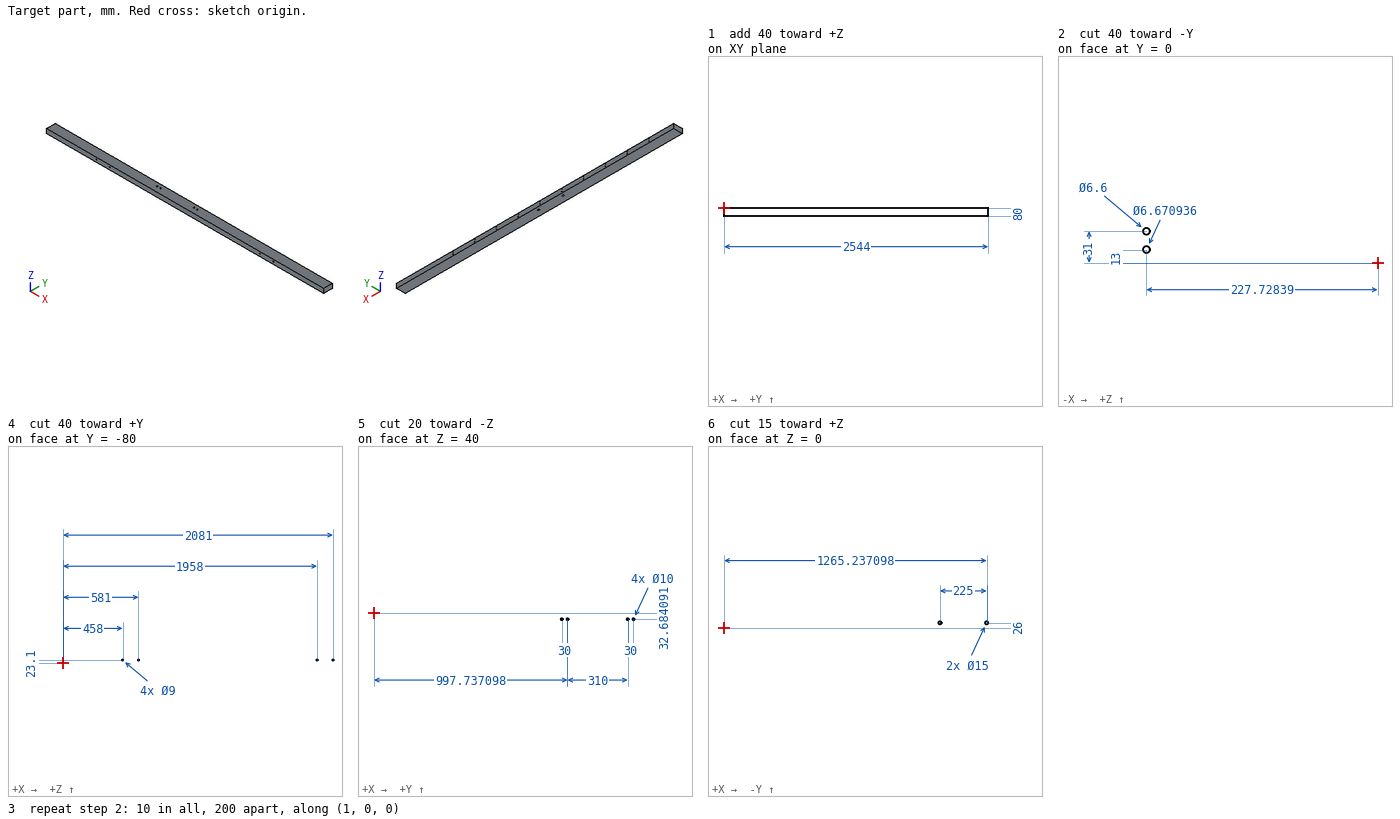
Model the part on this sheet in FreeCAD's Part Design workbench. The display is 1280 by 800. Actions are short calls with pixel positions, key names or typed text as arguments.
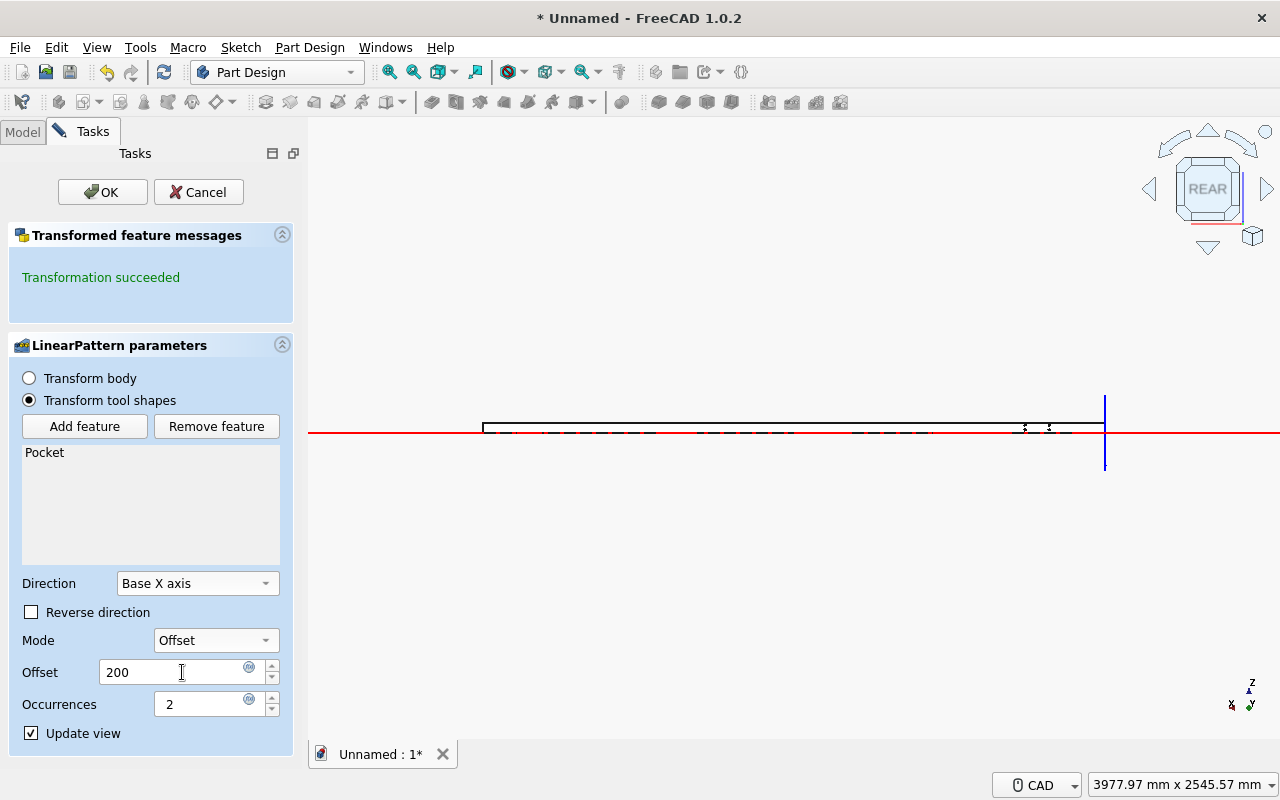
triple_click(209, 704)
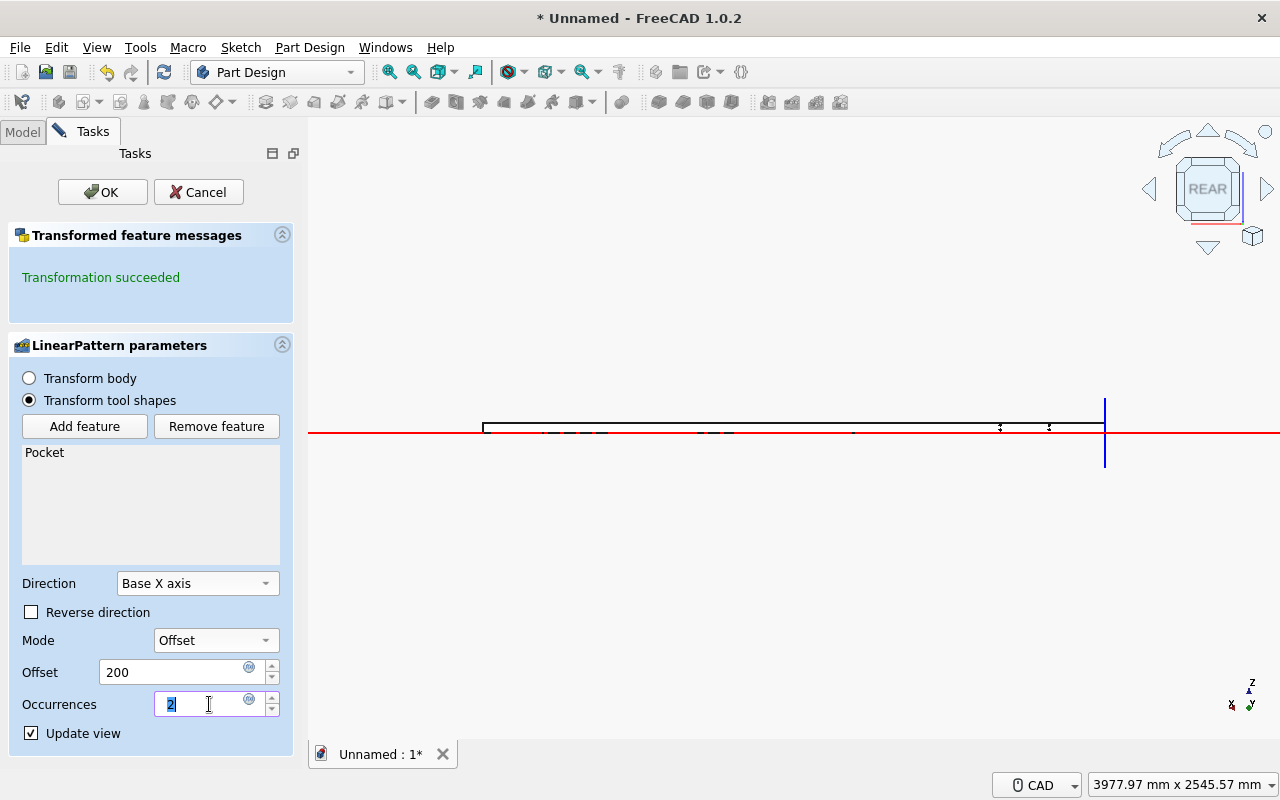
text(10)
key(Tab)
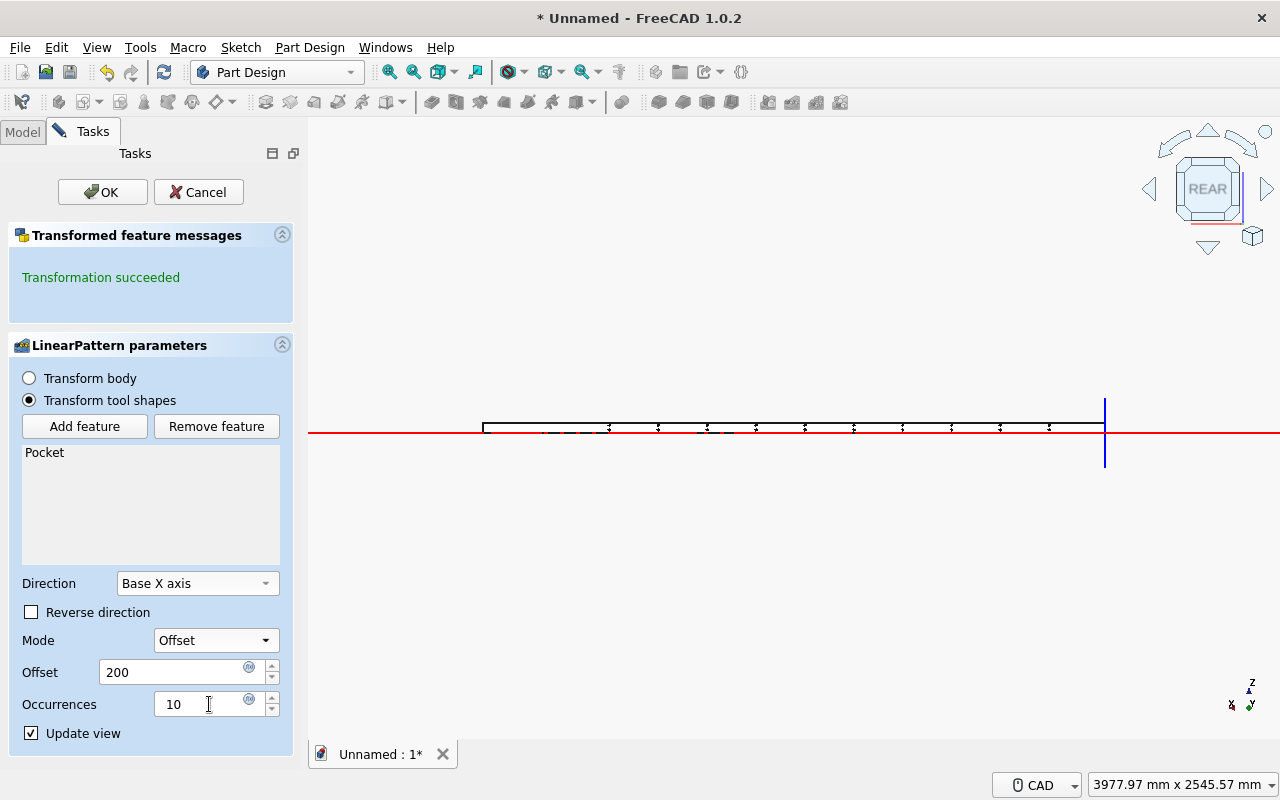
click(103, 192)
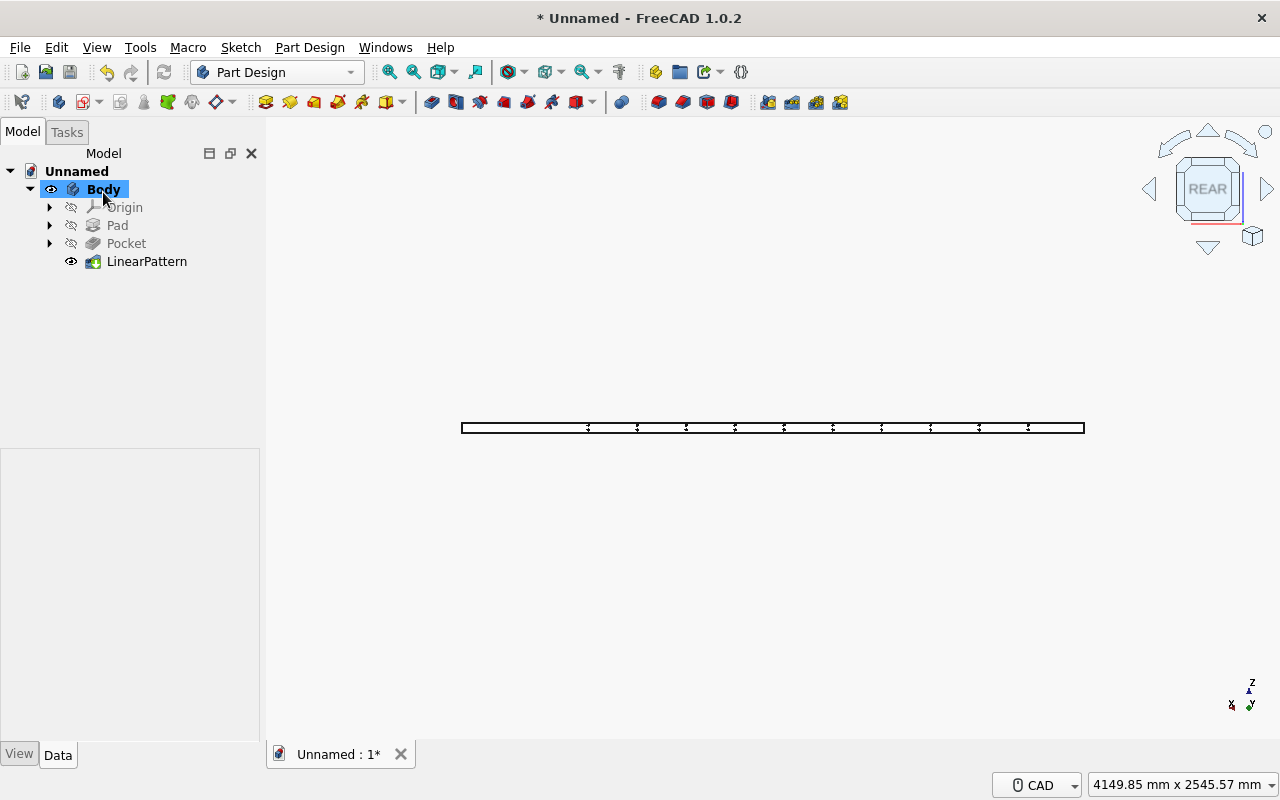
key(0)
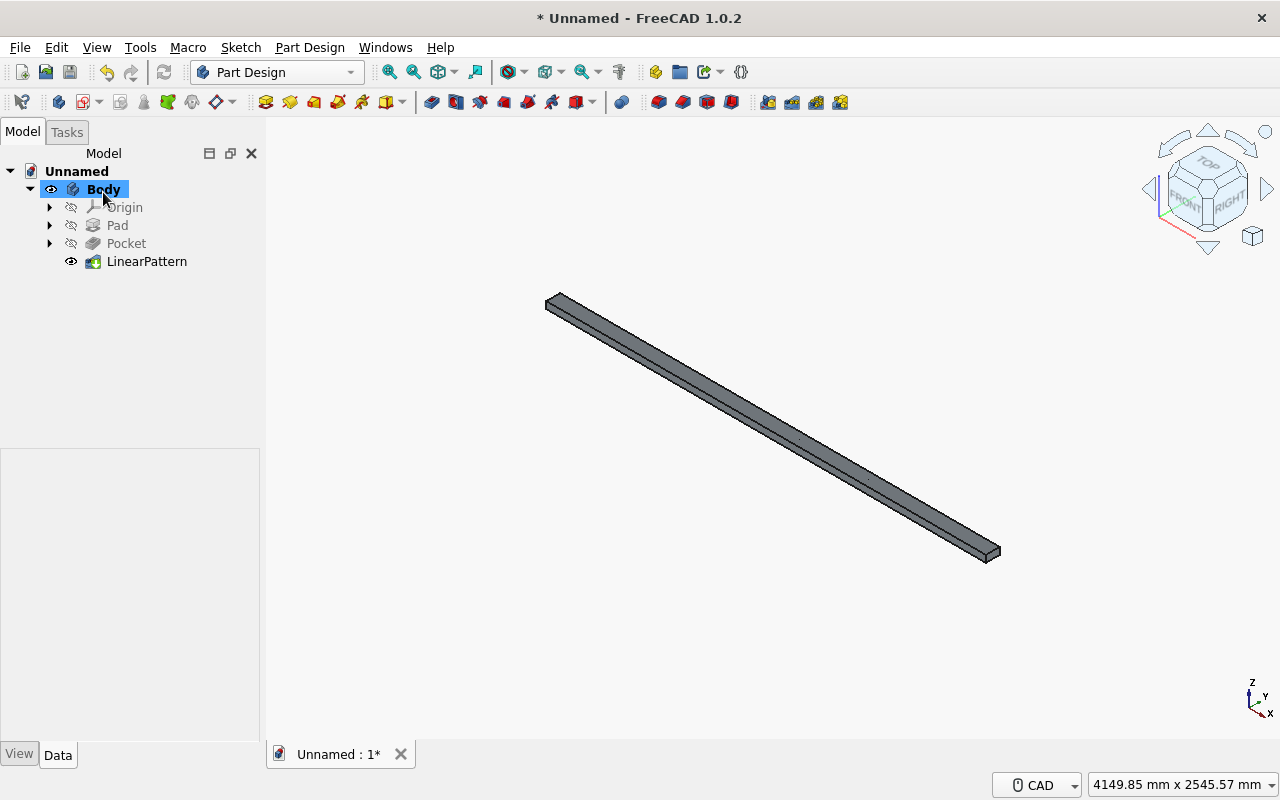
click(390, 72)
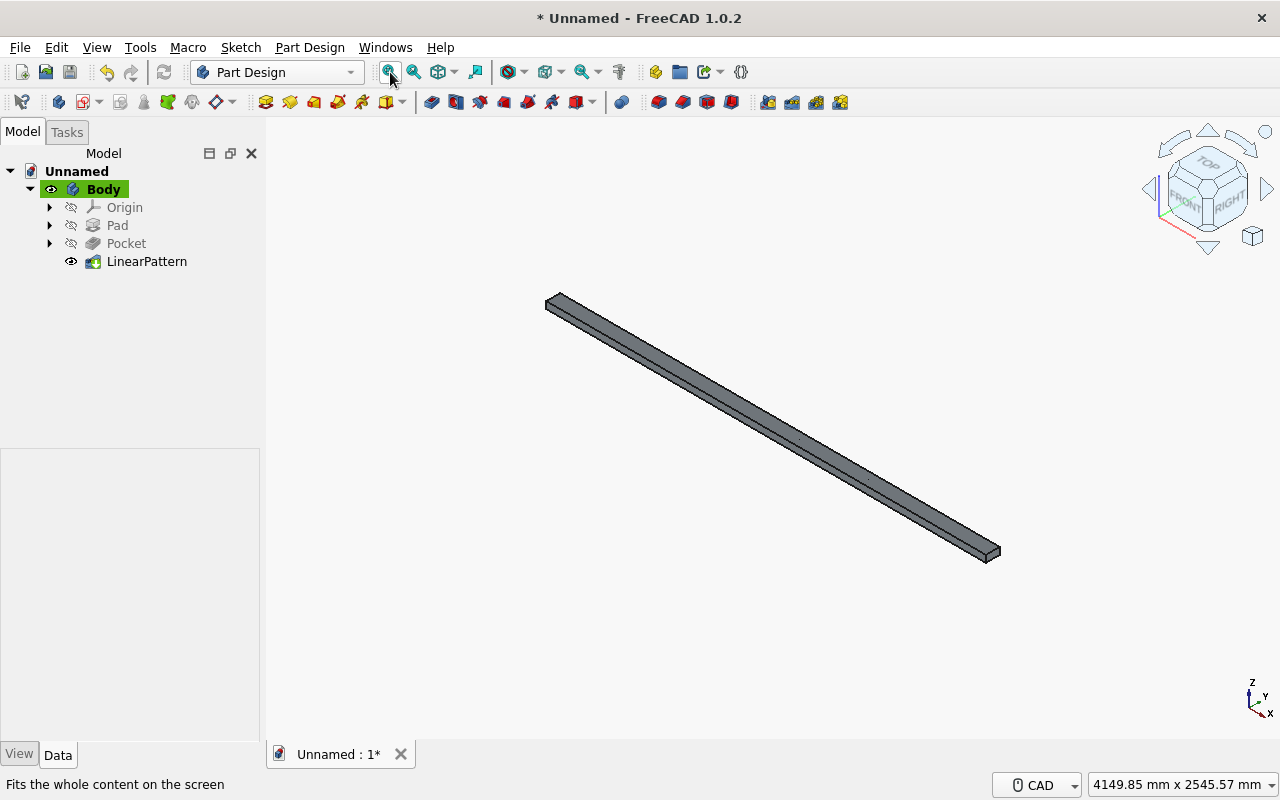
scroll(954, 540, up, 5)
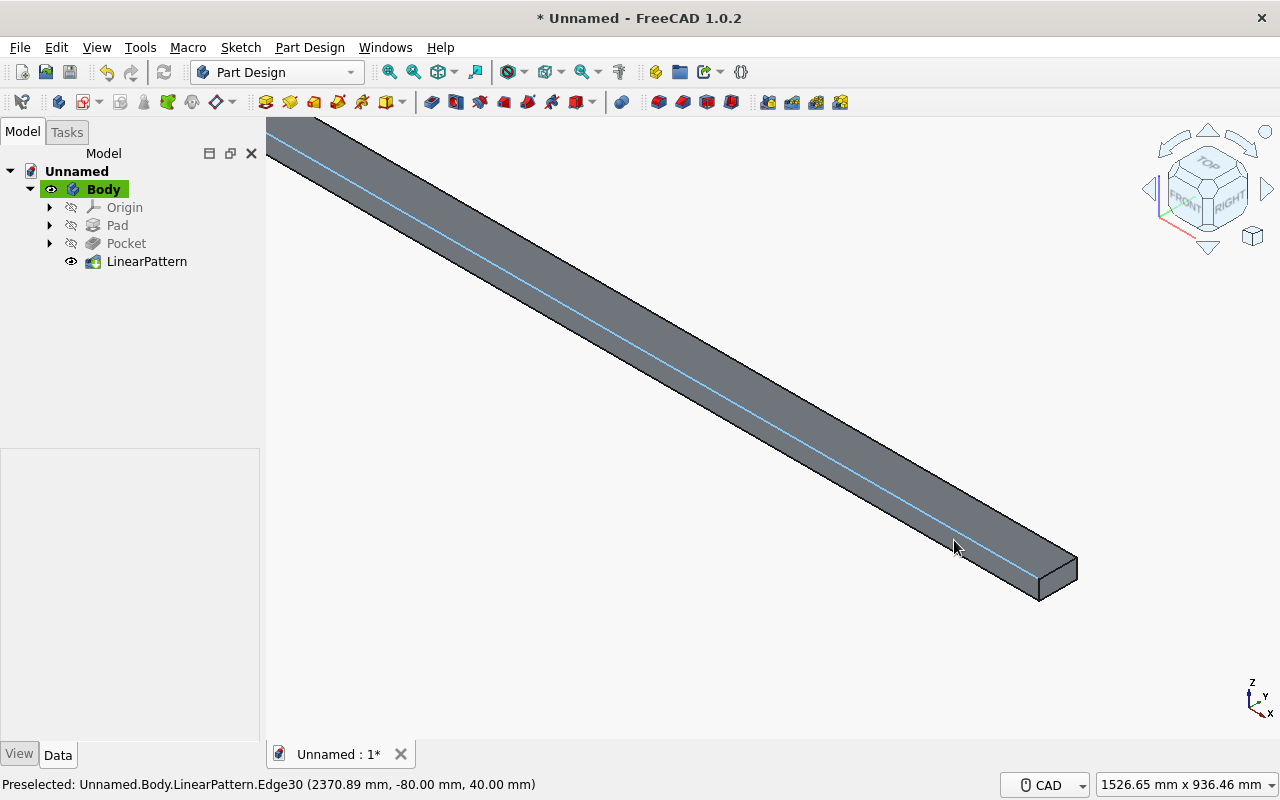
click(954, 540)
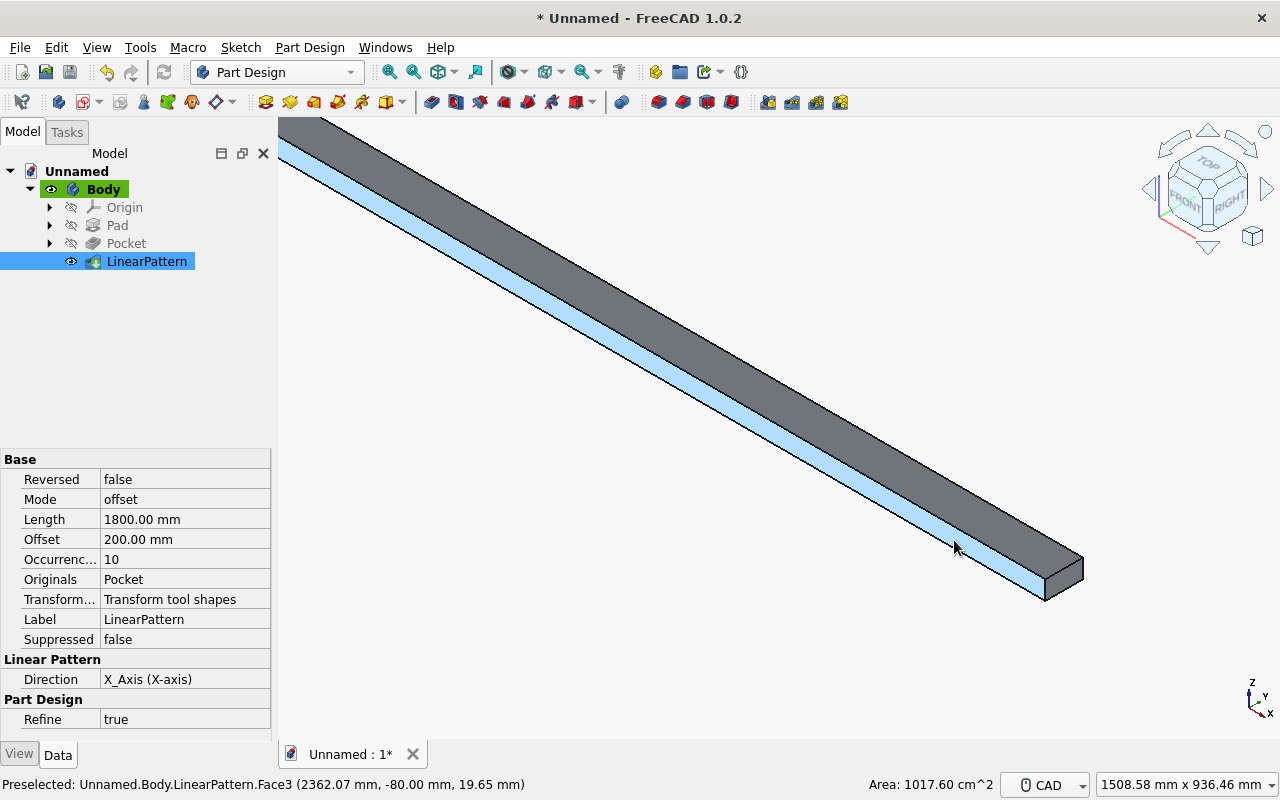
click(84, 102)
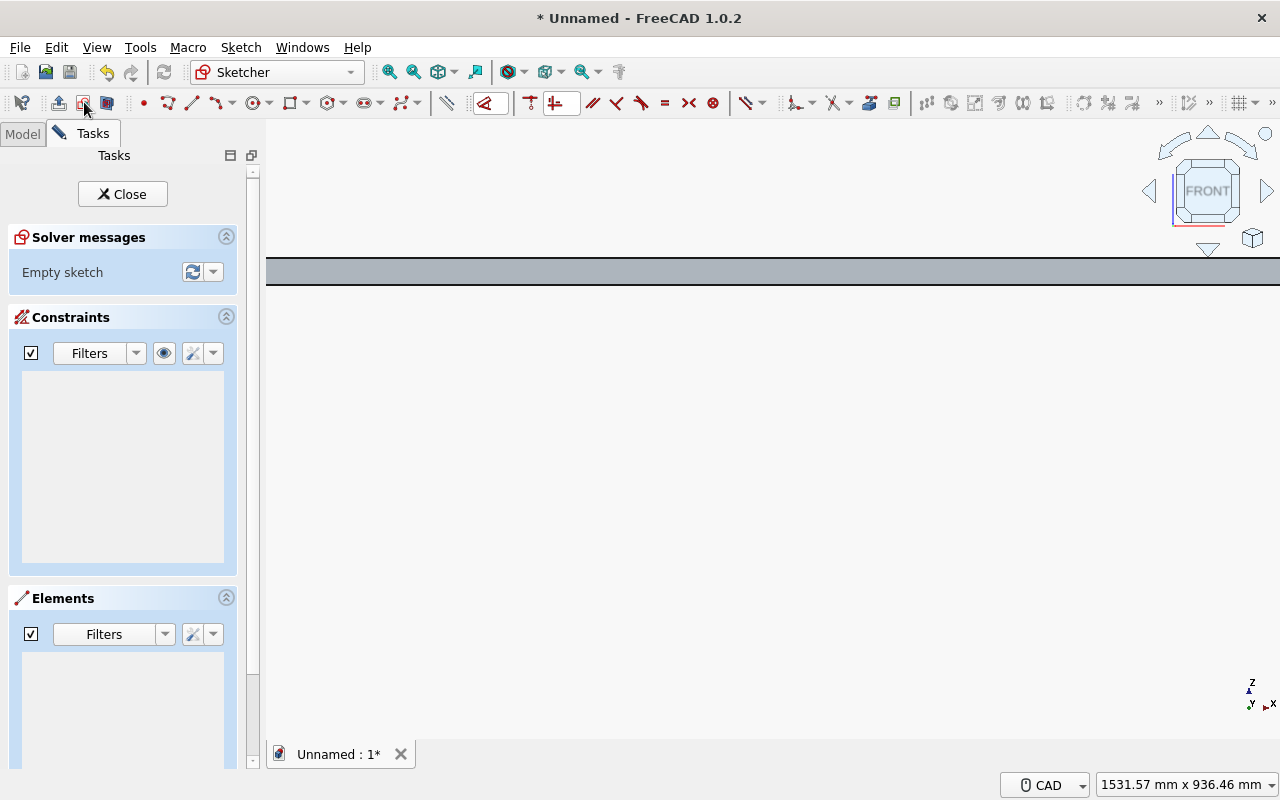
scroll(1016, 554, down, 4)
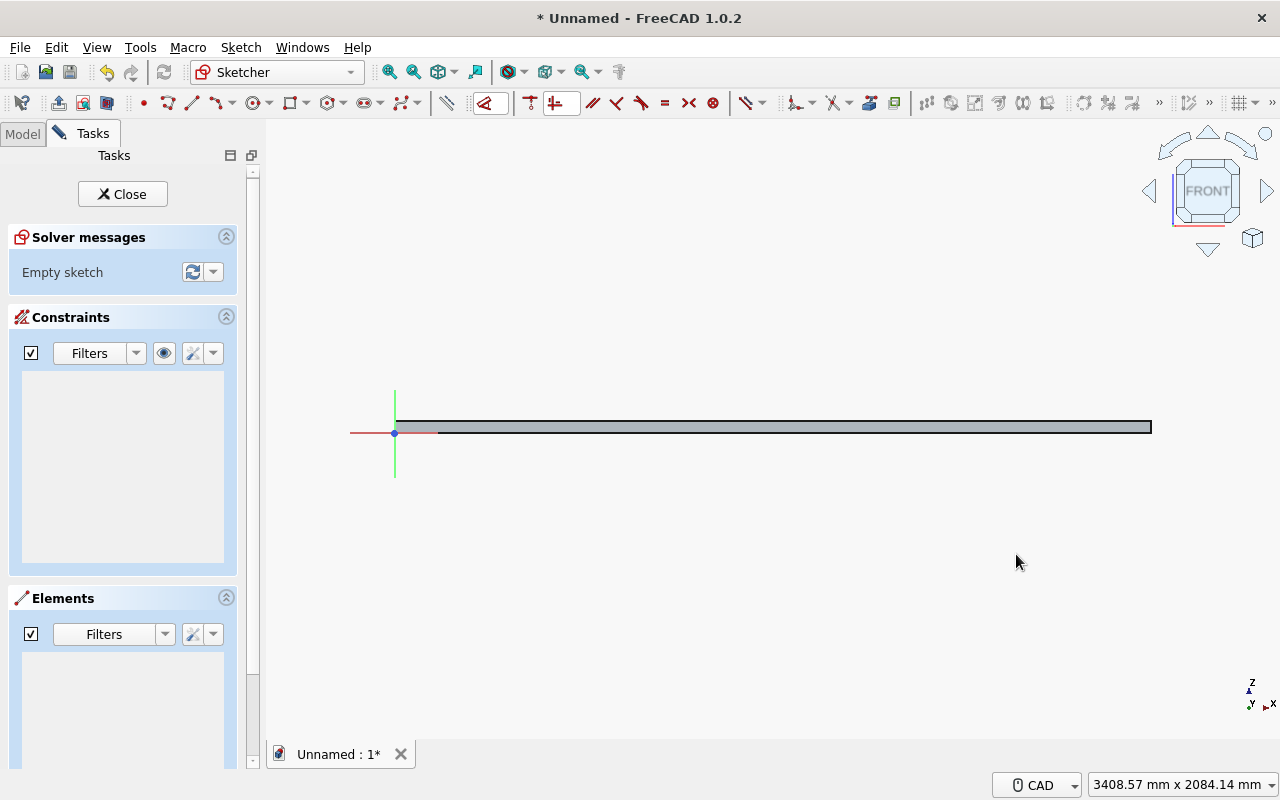
key(g)
key(c)